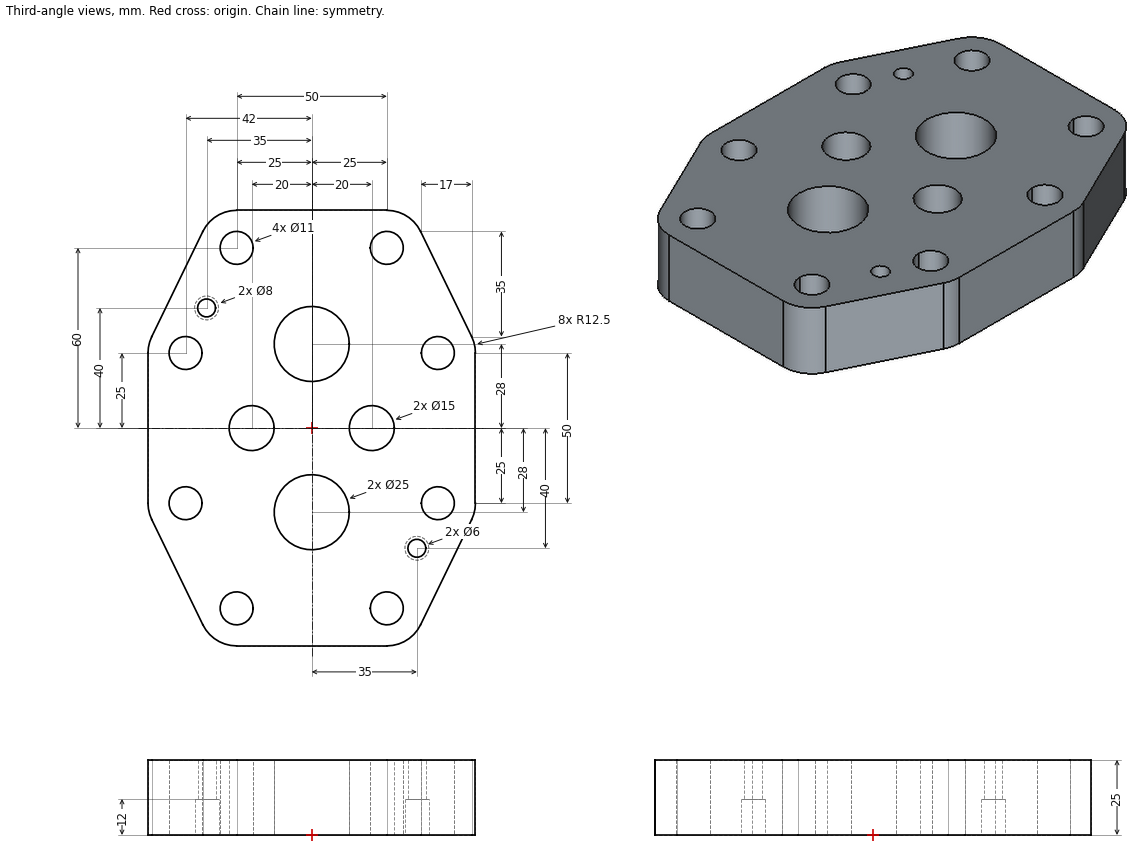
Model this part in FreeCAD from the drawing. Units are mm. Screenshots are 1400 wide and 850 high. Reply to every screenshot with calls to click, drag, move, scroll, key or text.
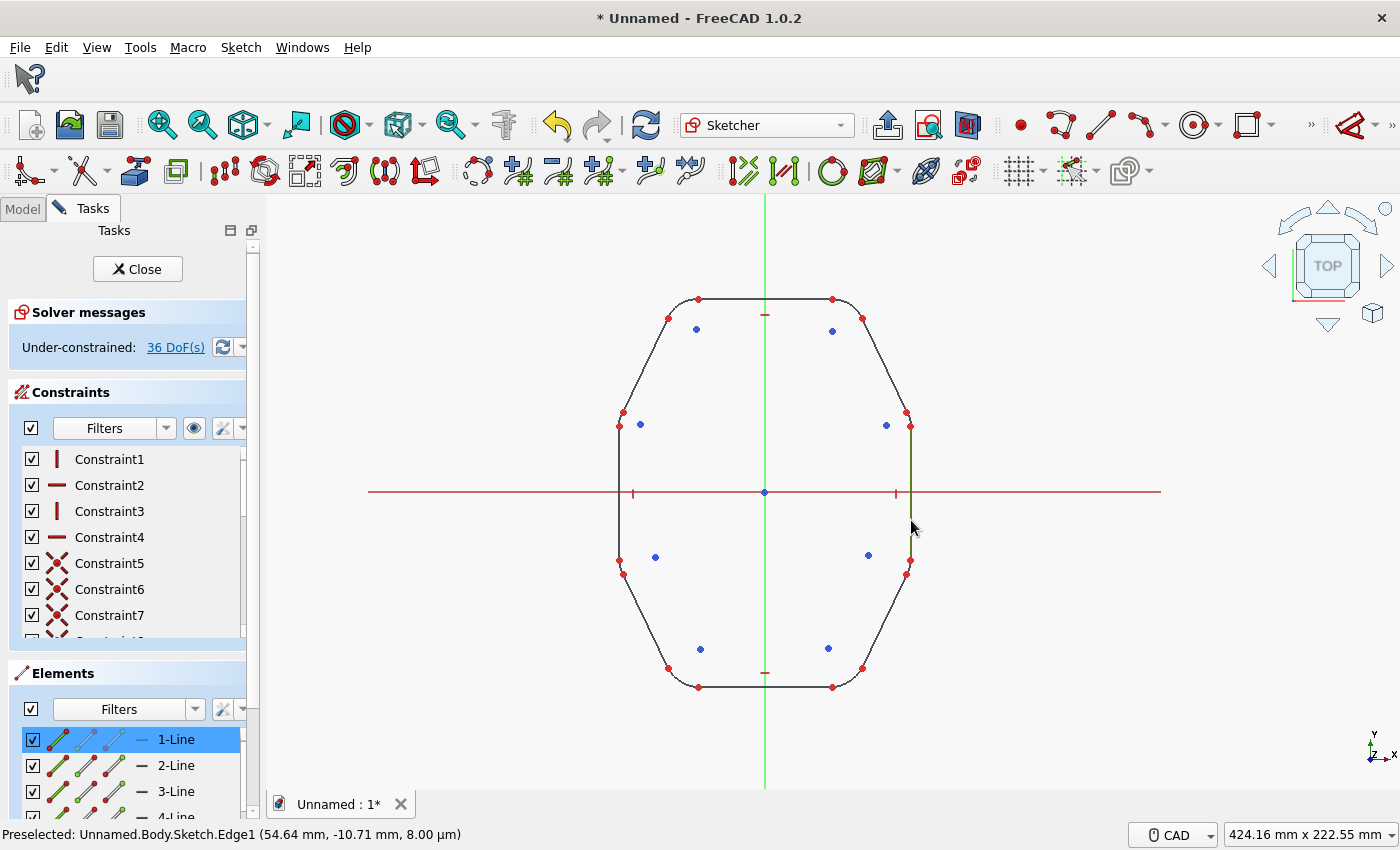
scroll(910, 419, up, 4)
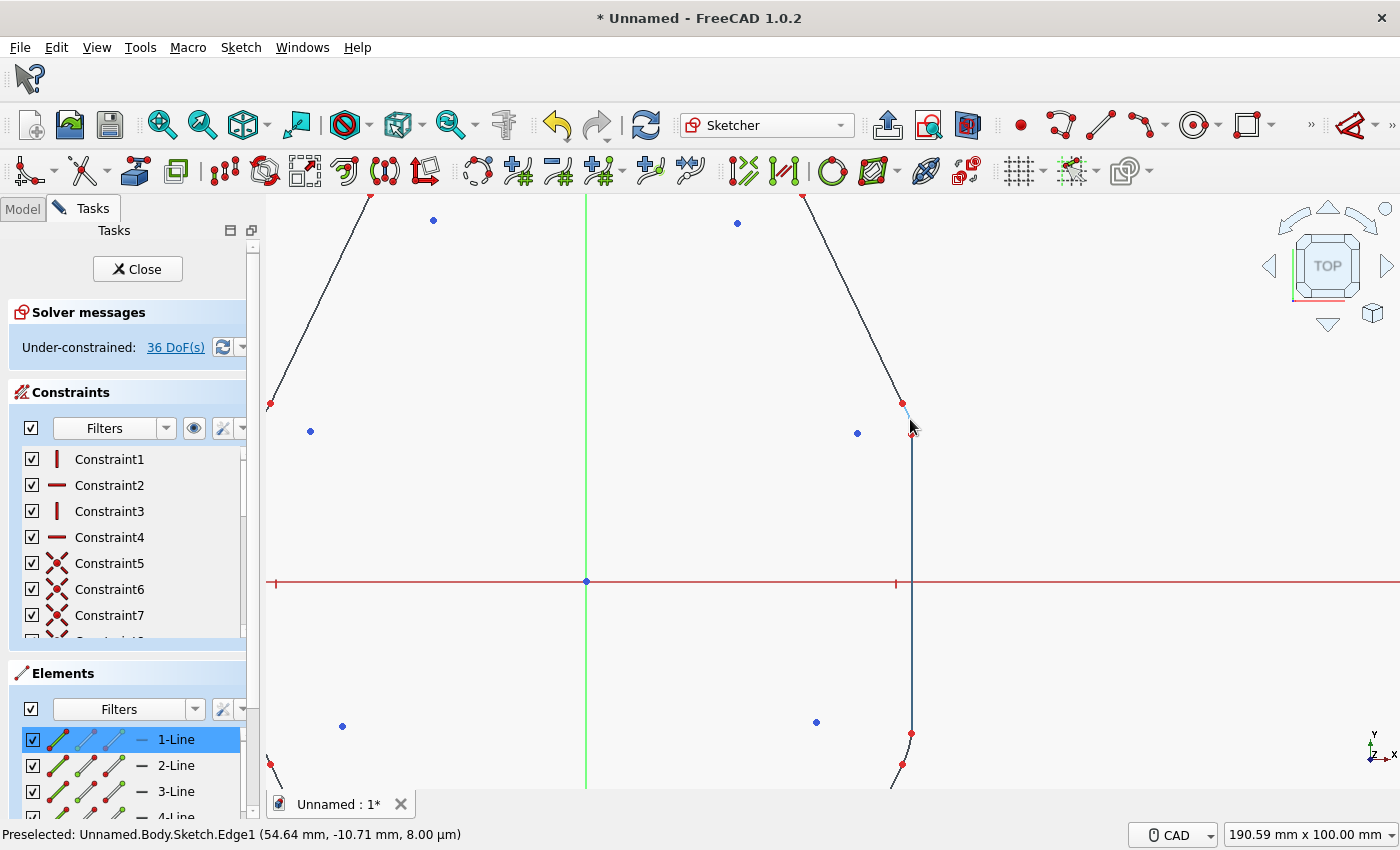
click(909, 419)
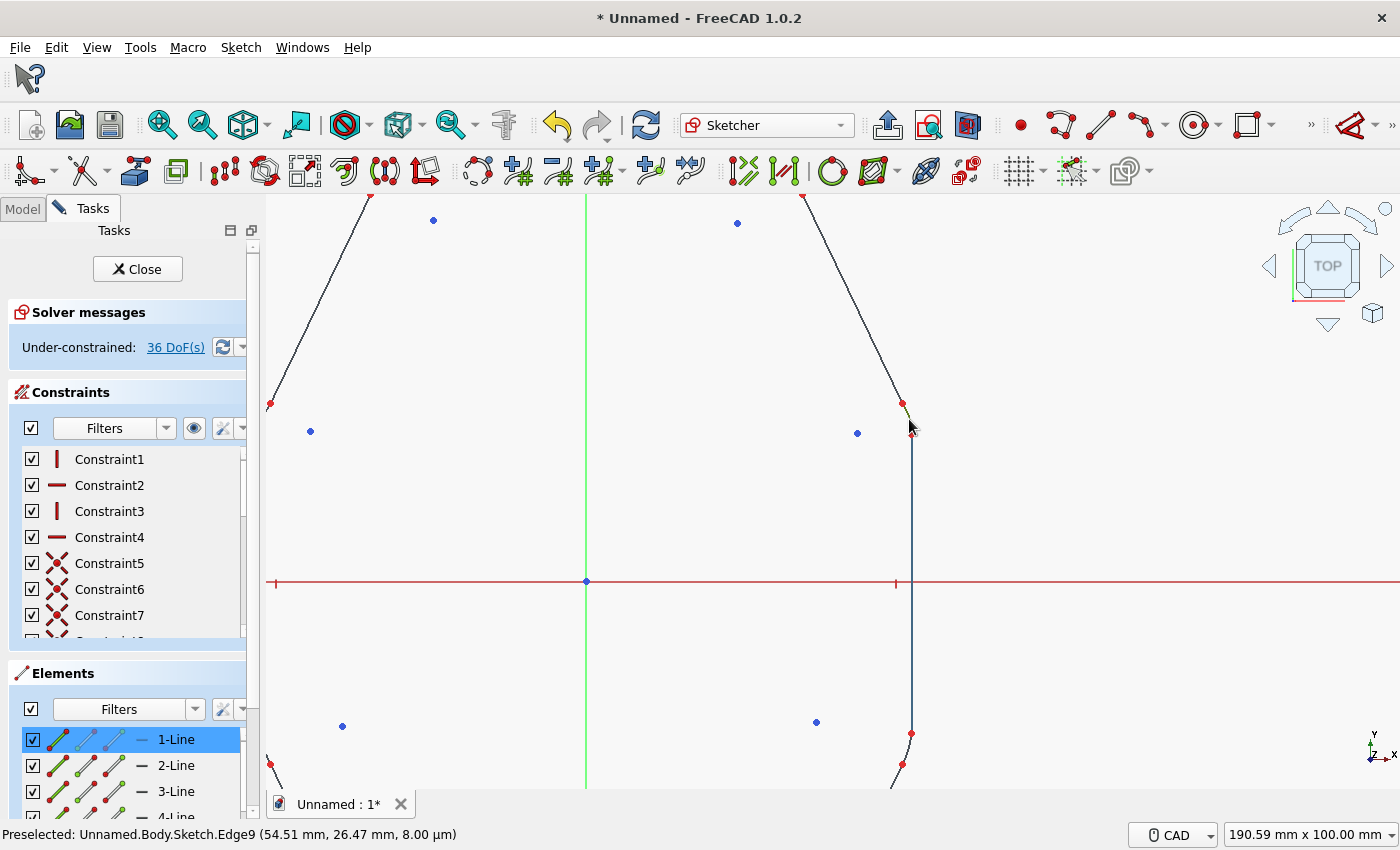
key(t)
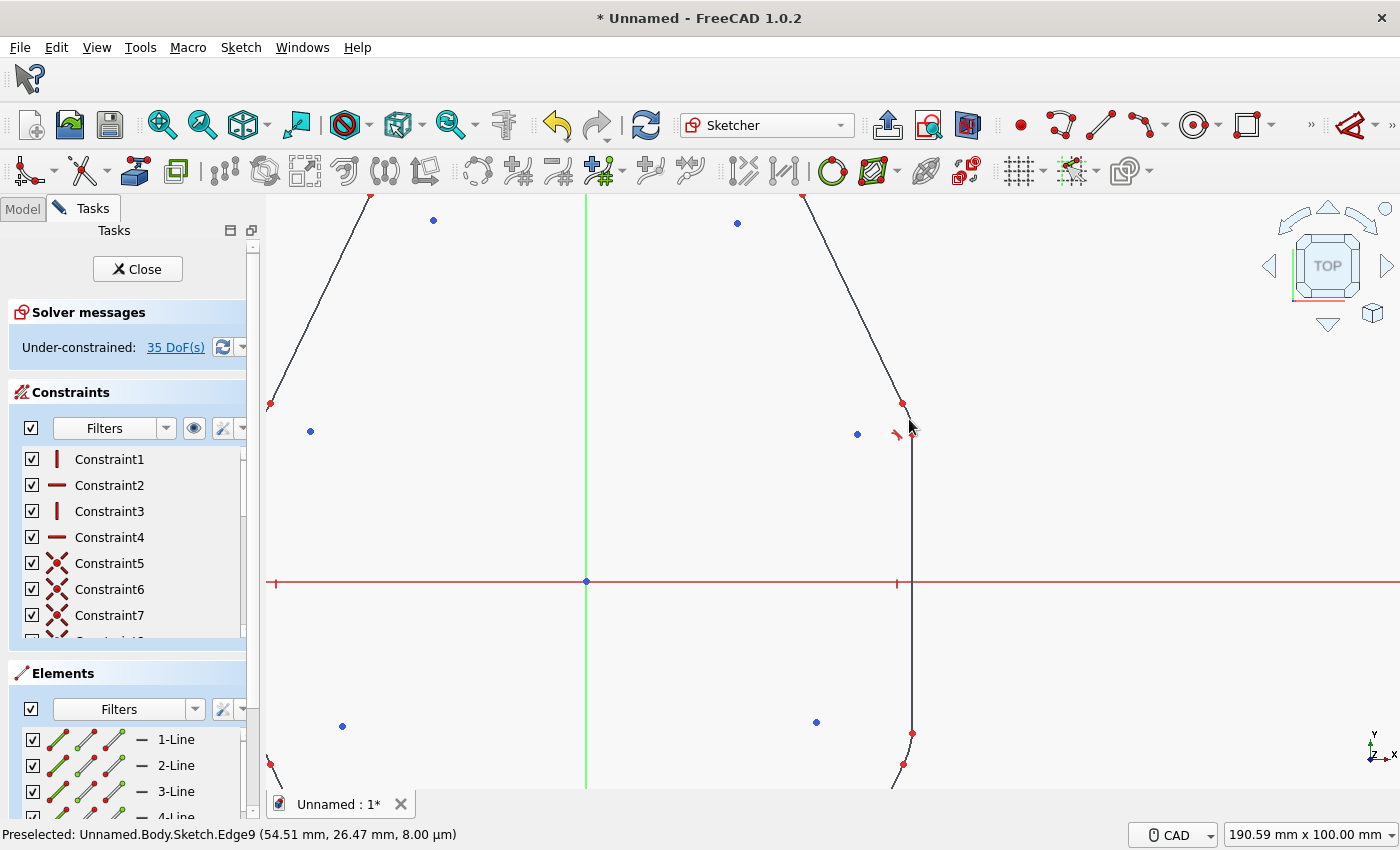
click(912, 644)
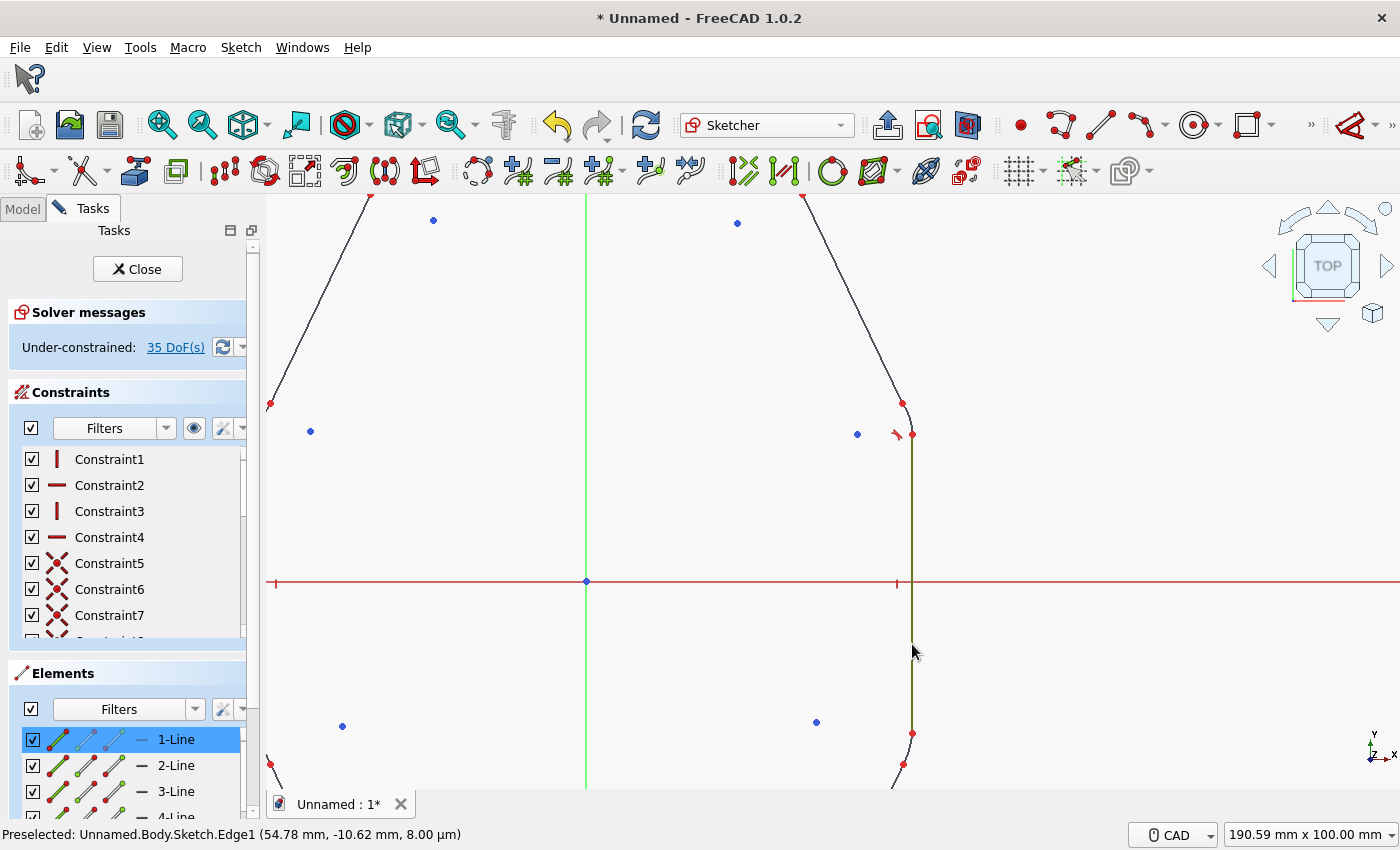
scroll(907, 755, up, 2)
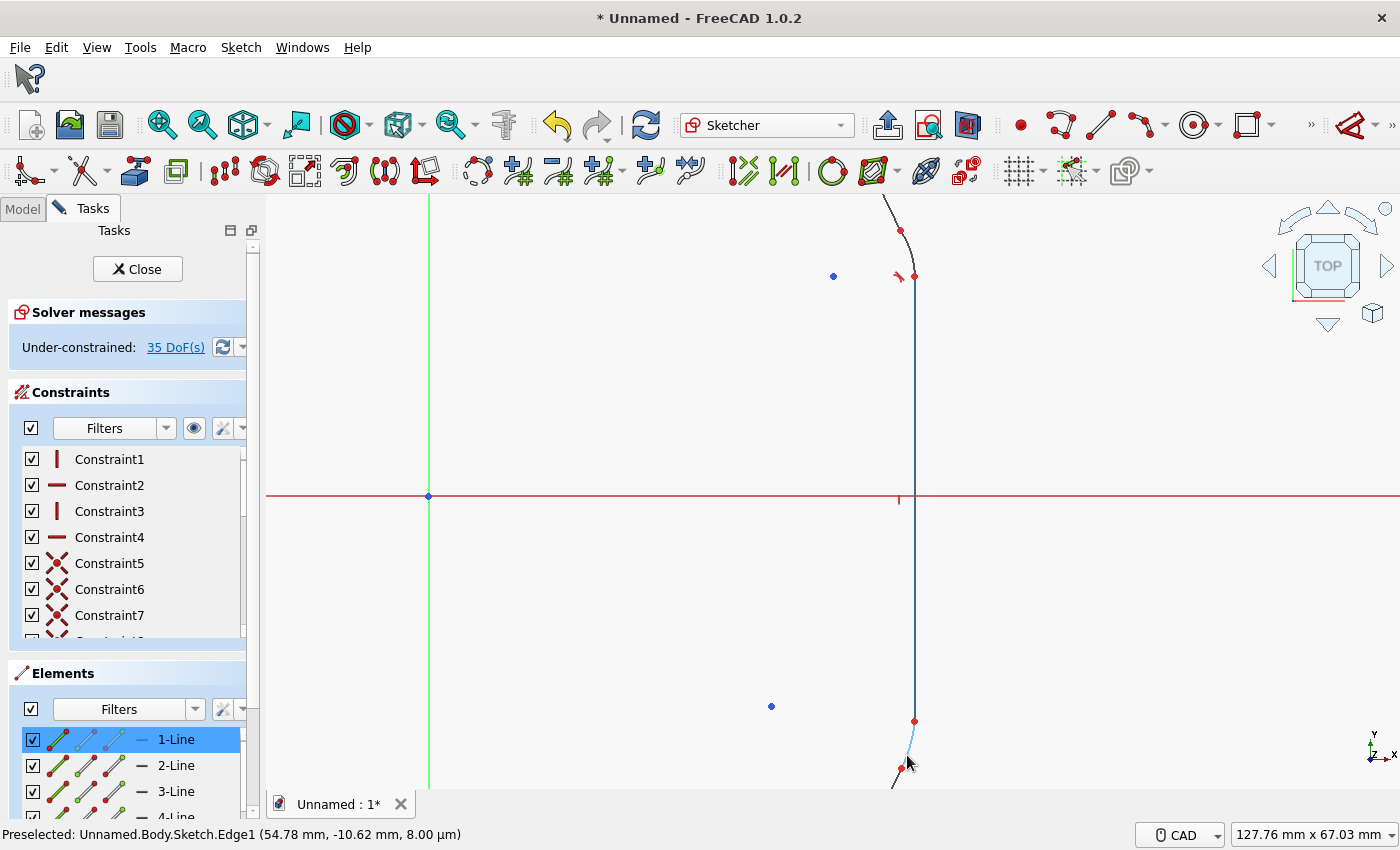
click(907, 755)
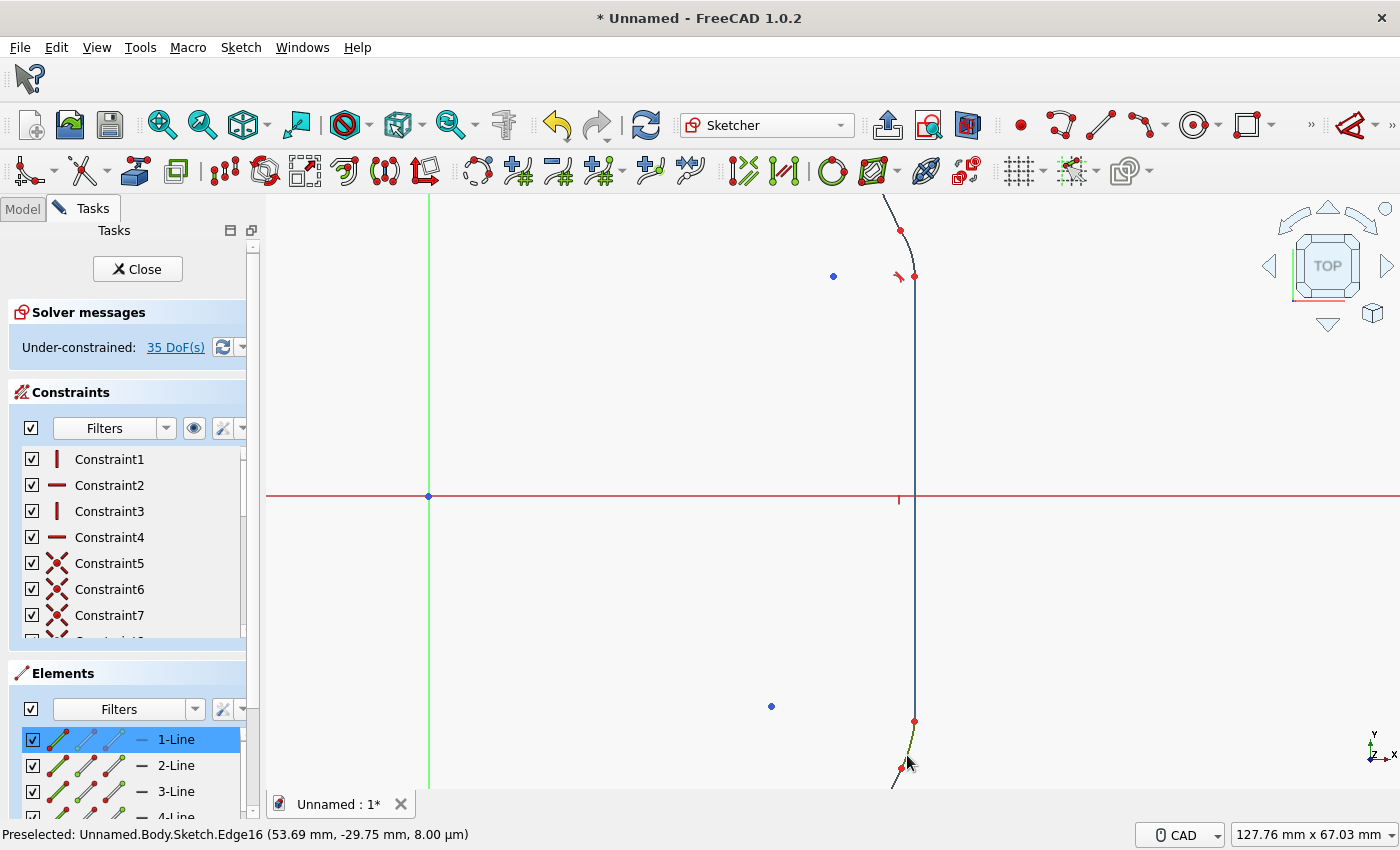
key(t)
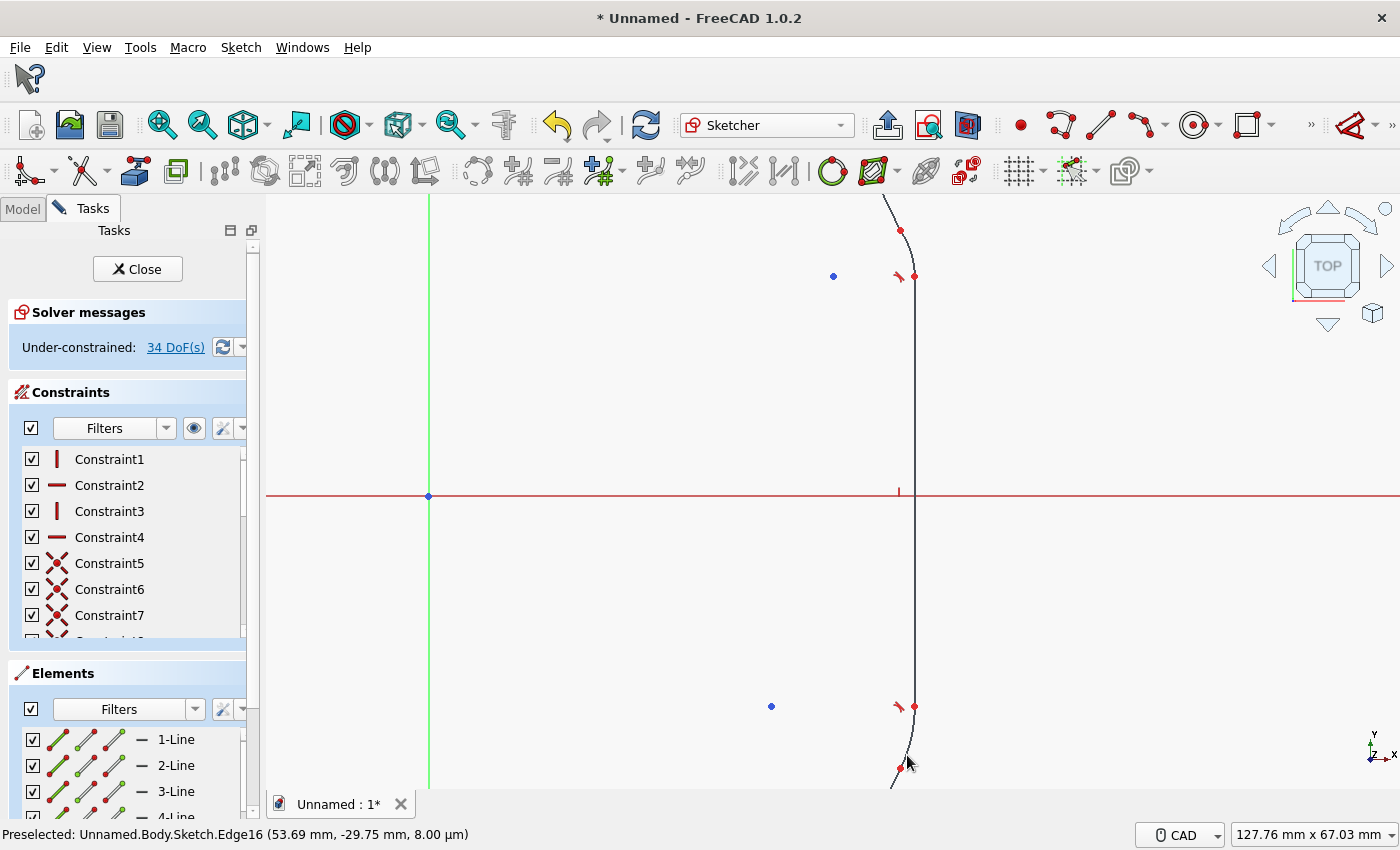
scroll(909, 489, down, 6)